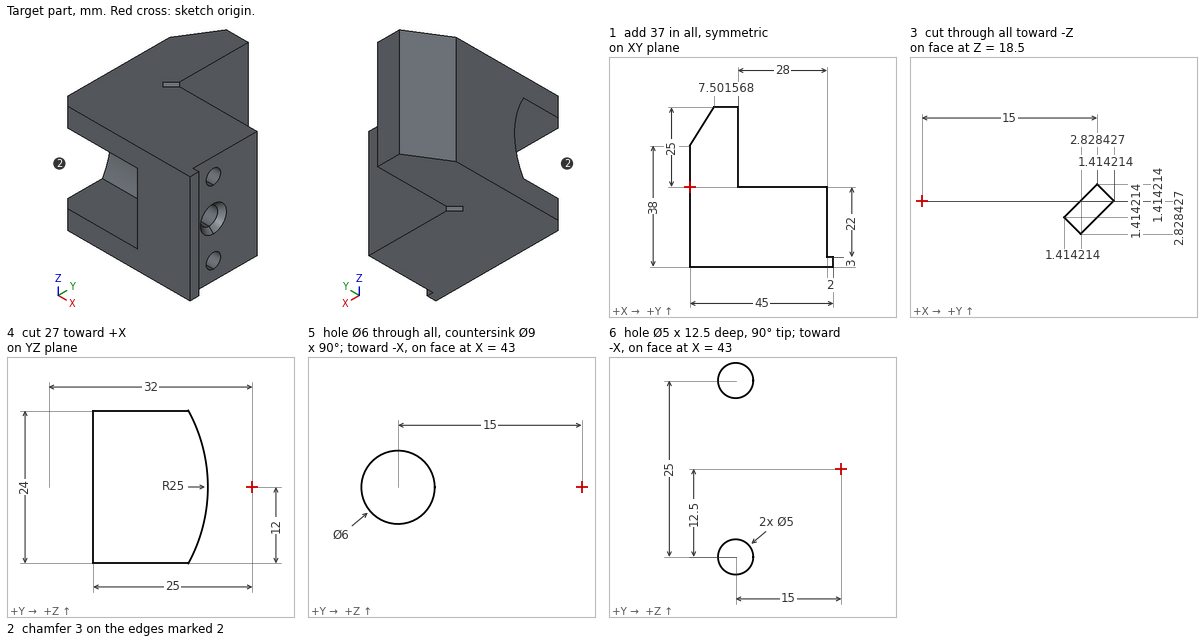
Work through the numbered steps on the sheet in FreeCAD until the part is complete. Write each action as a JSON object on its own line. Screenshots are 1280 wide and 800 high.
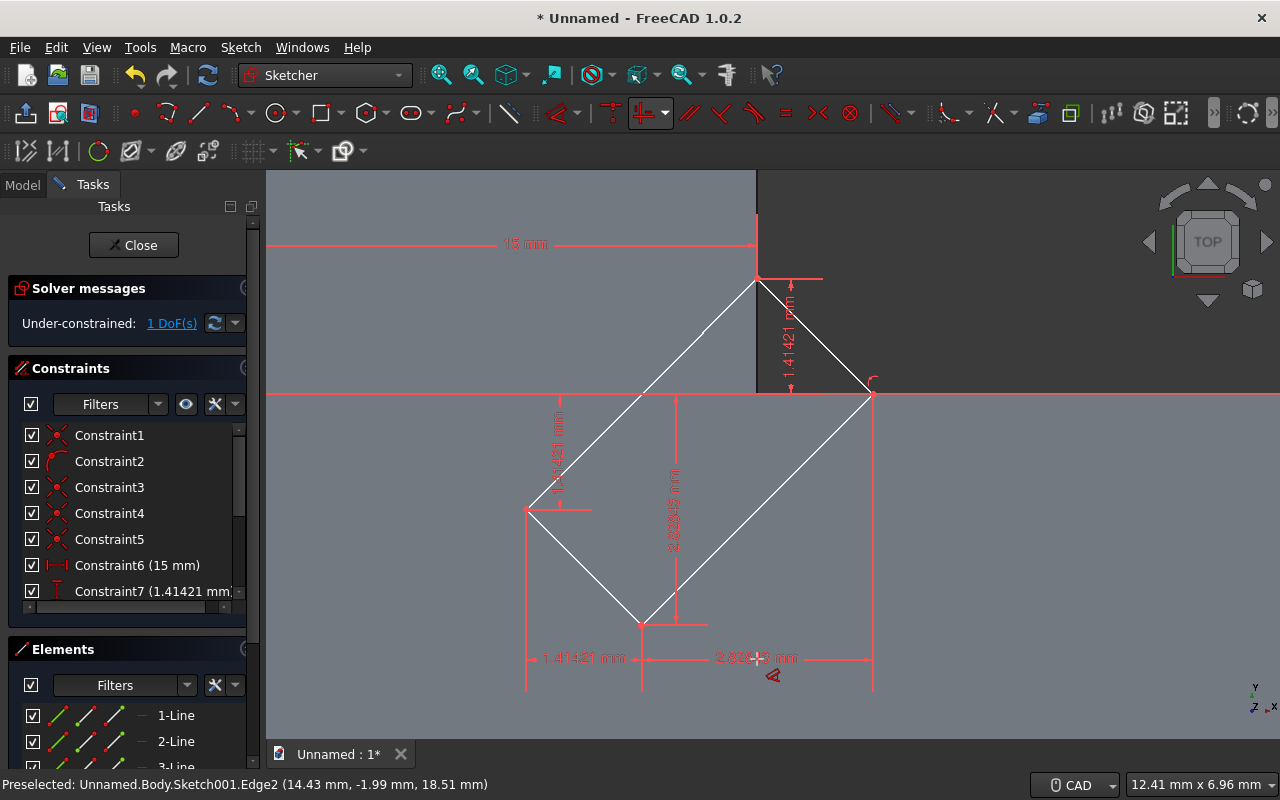
{"action": "left_click", "coordinate": [838, 360]}
{"action": "left_click", "coordinate": [815, 245]}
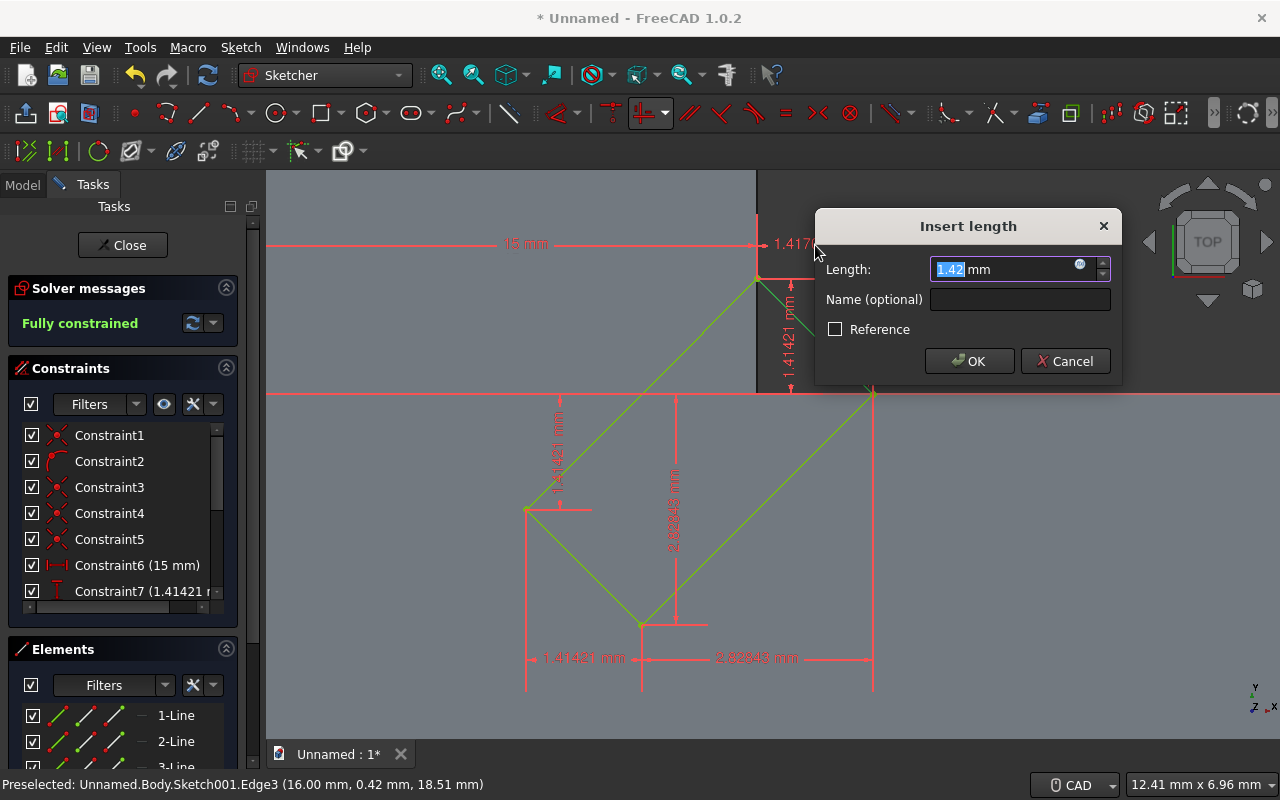
{"action": "type", "text": "1.414214"}
{"action": "key", "text": "Return"}
{"action": "key", "text": "Escape"}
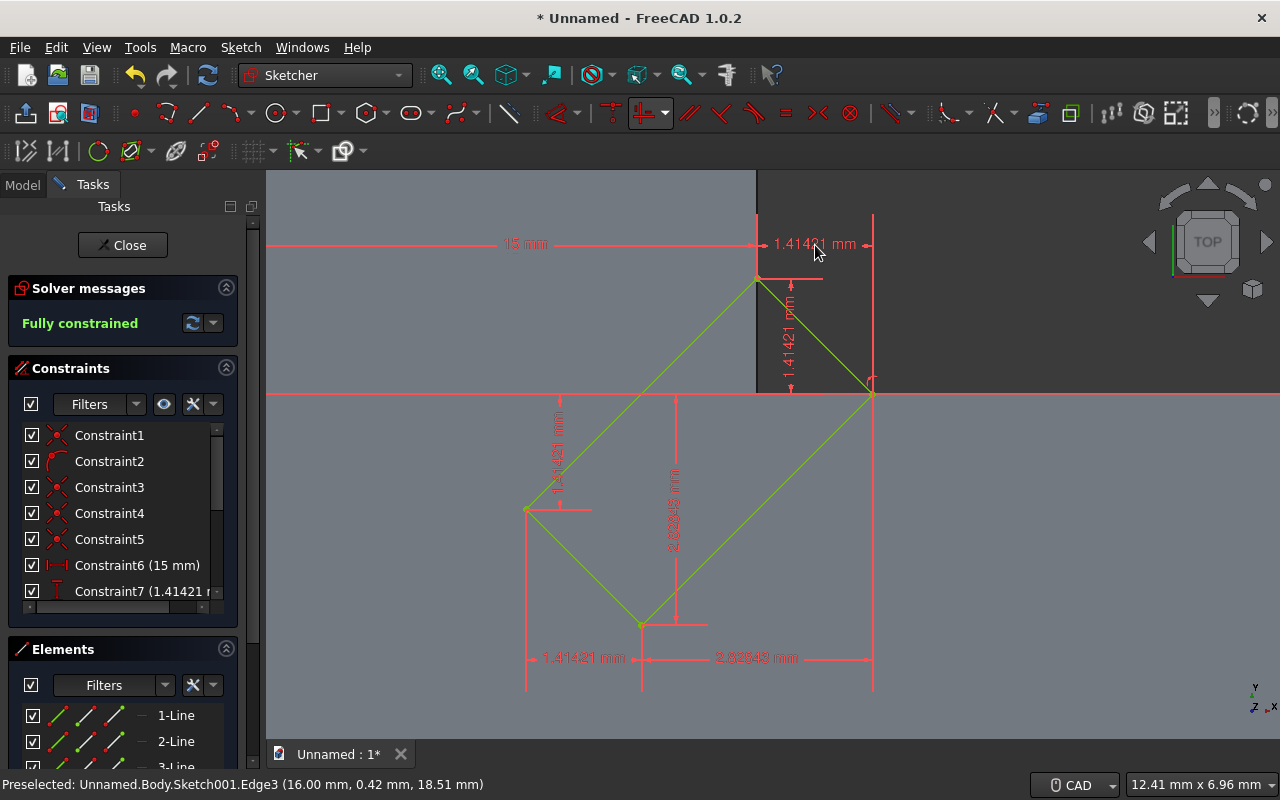
{"action": "left_click", "coordinate": [123, 245]}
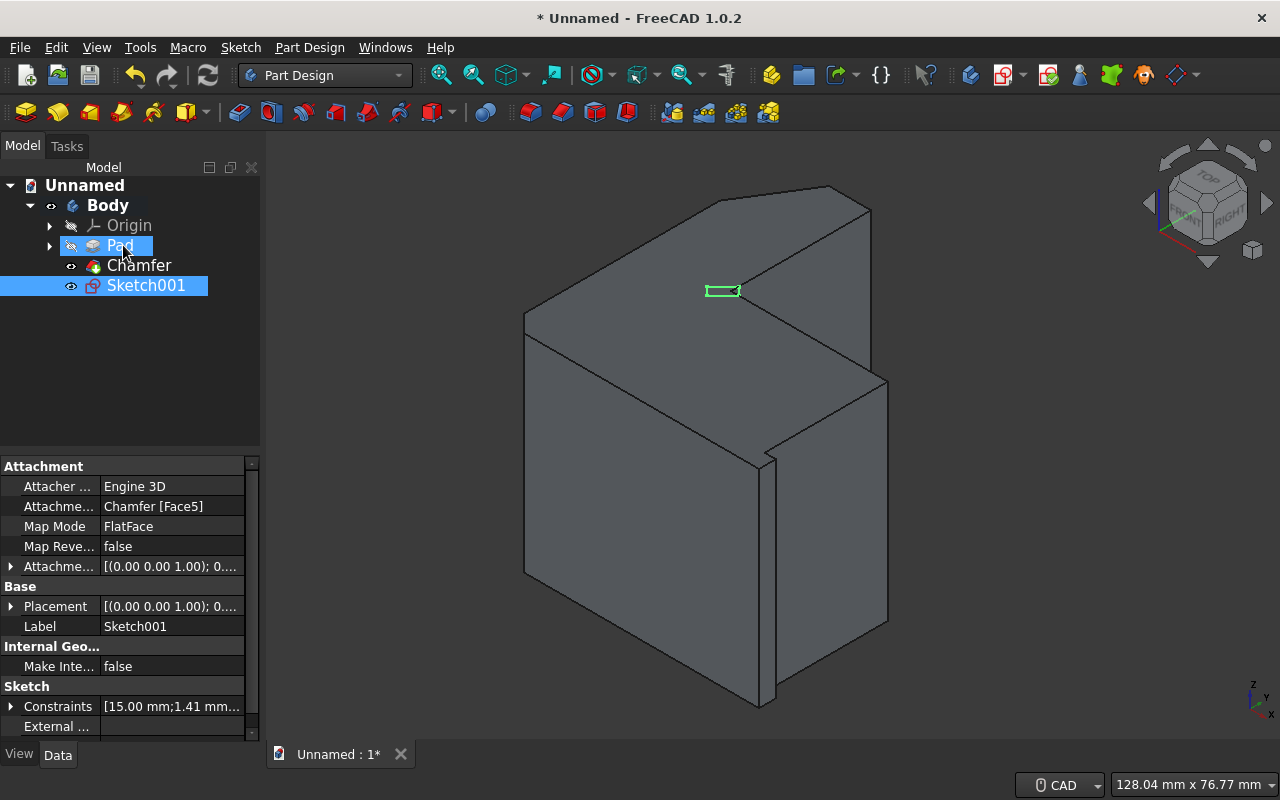
{"action": "left_click", "coordinate": [240, 112]}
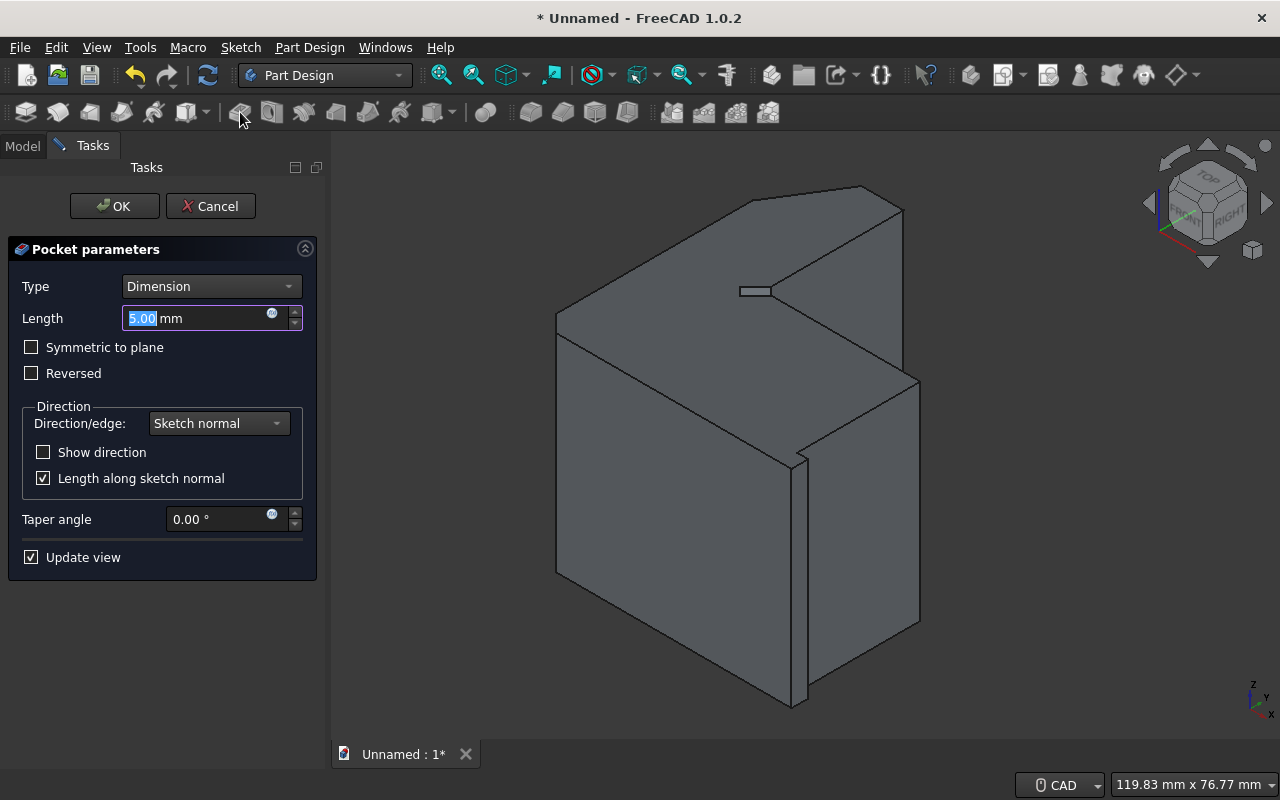
{"action": "left_click", "coordinate": [212, 286]}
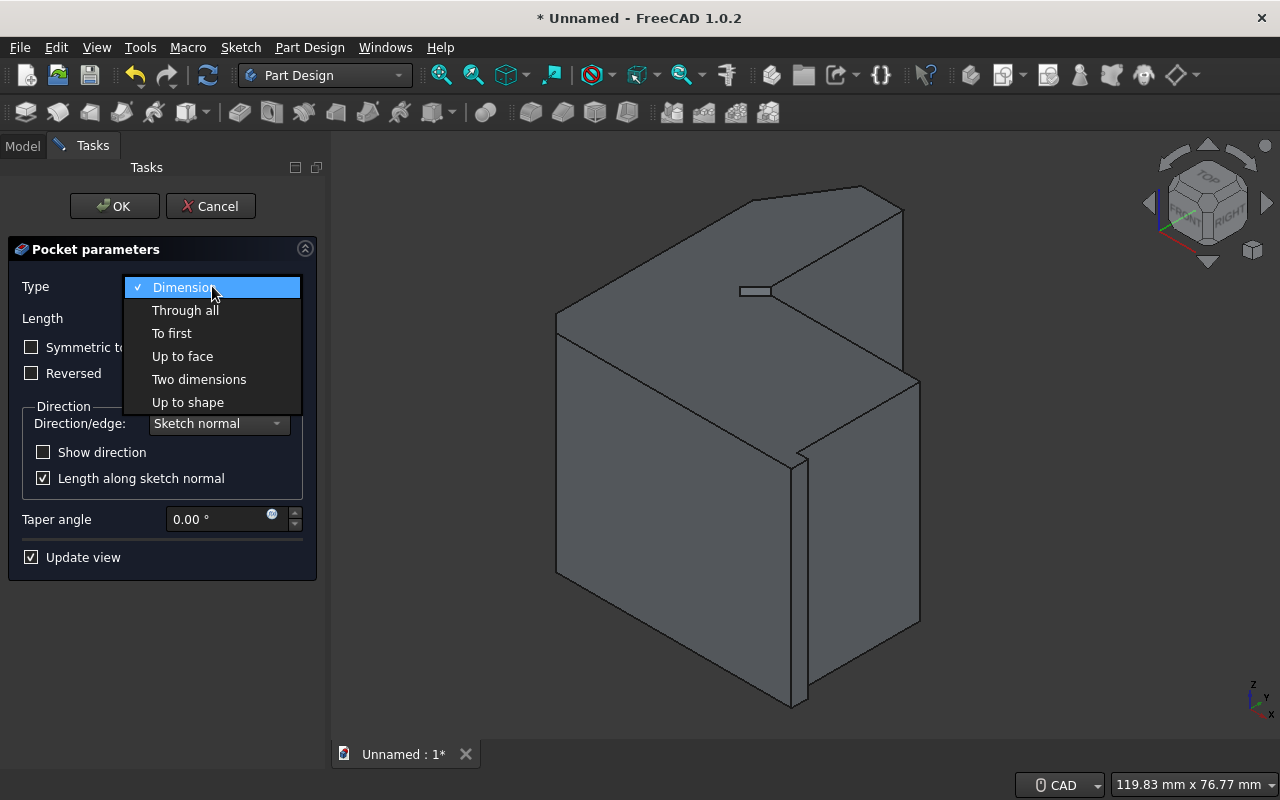
{"action": "left_click", "coordinate": [212, 310]}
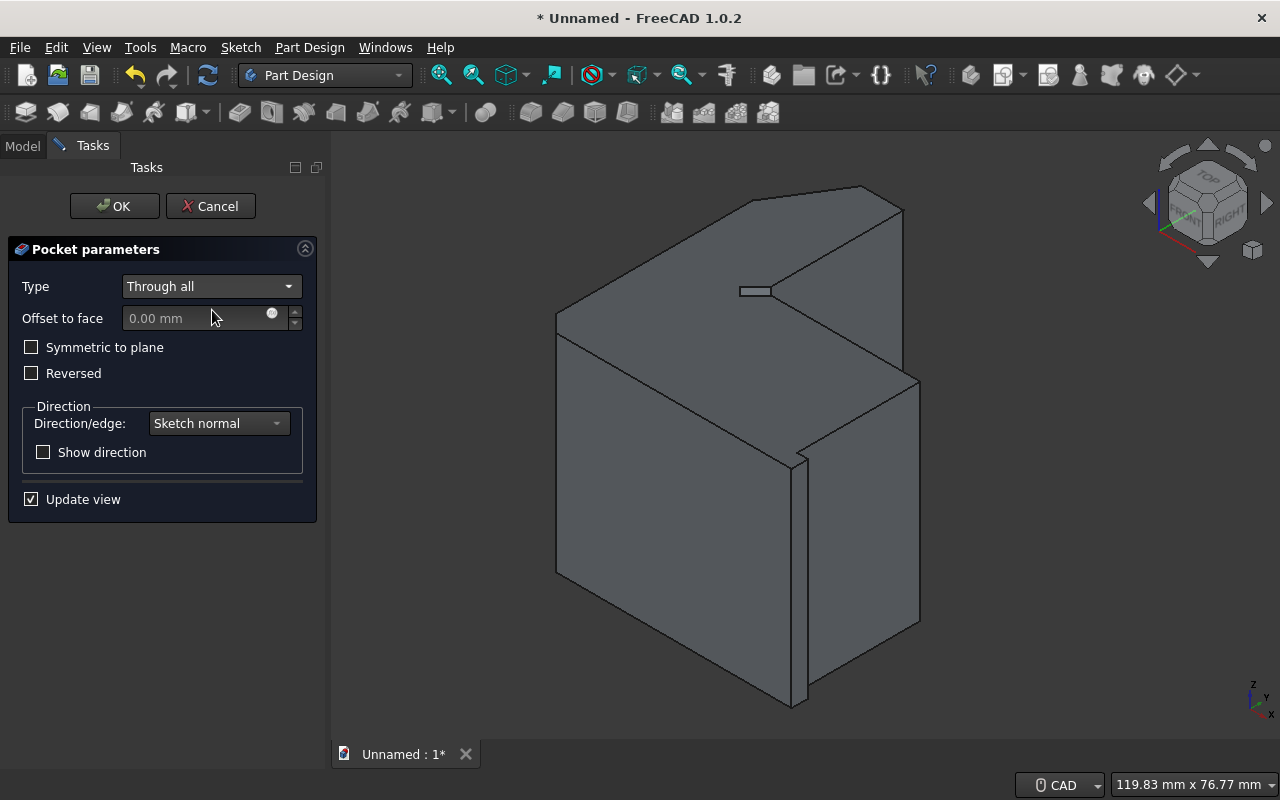
{"action": "left_click", "coordinate": [115, 206]}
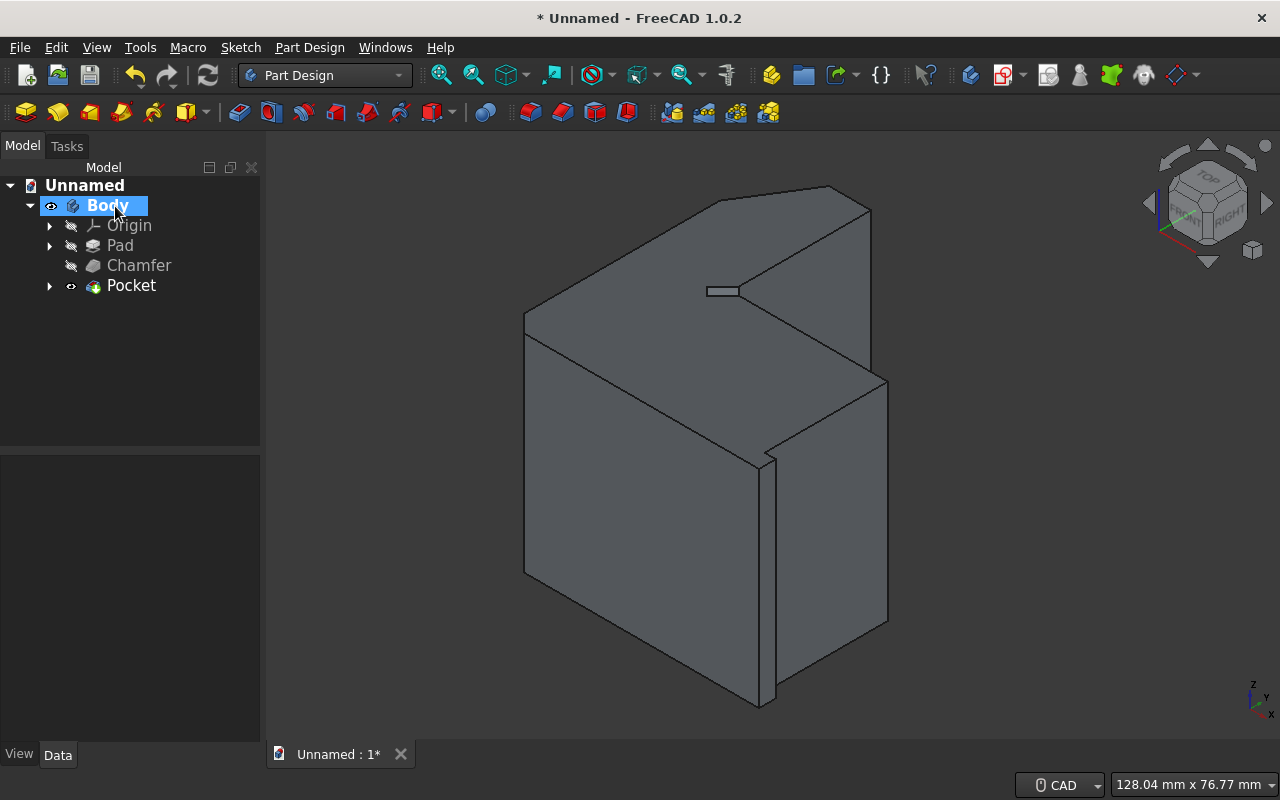
{"action": "left_click", "coordinate": [1004, 76]}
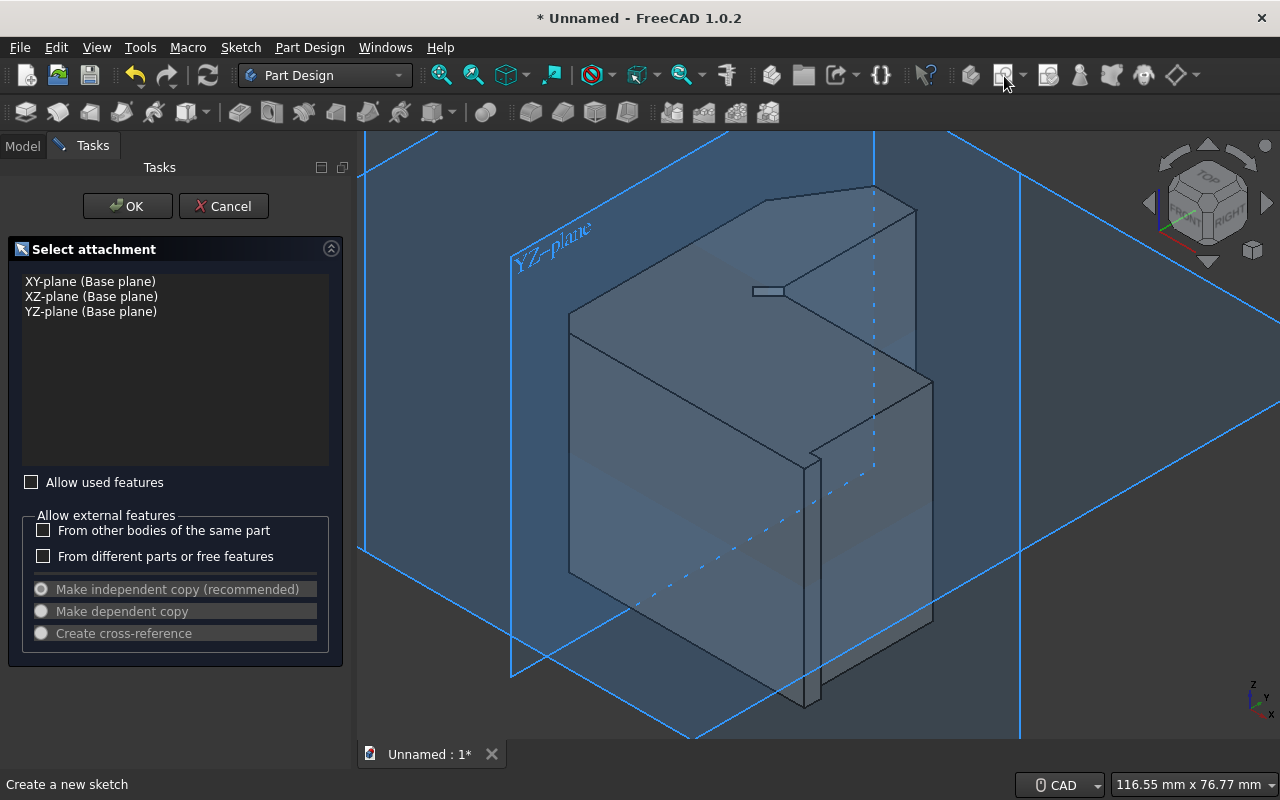
{"action": "left_click", "coordinate": [82, 312]}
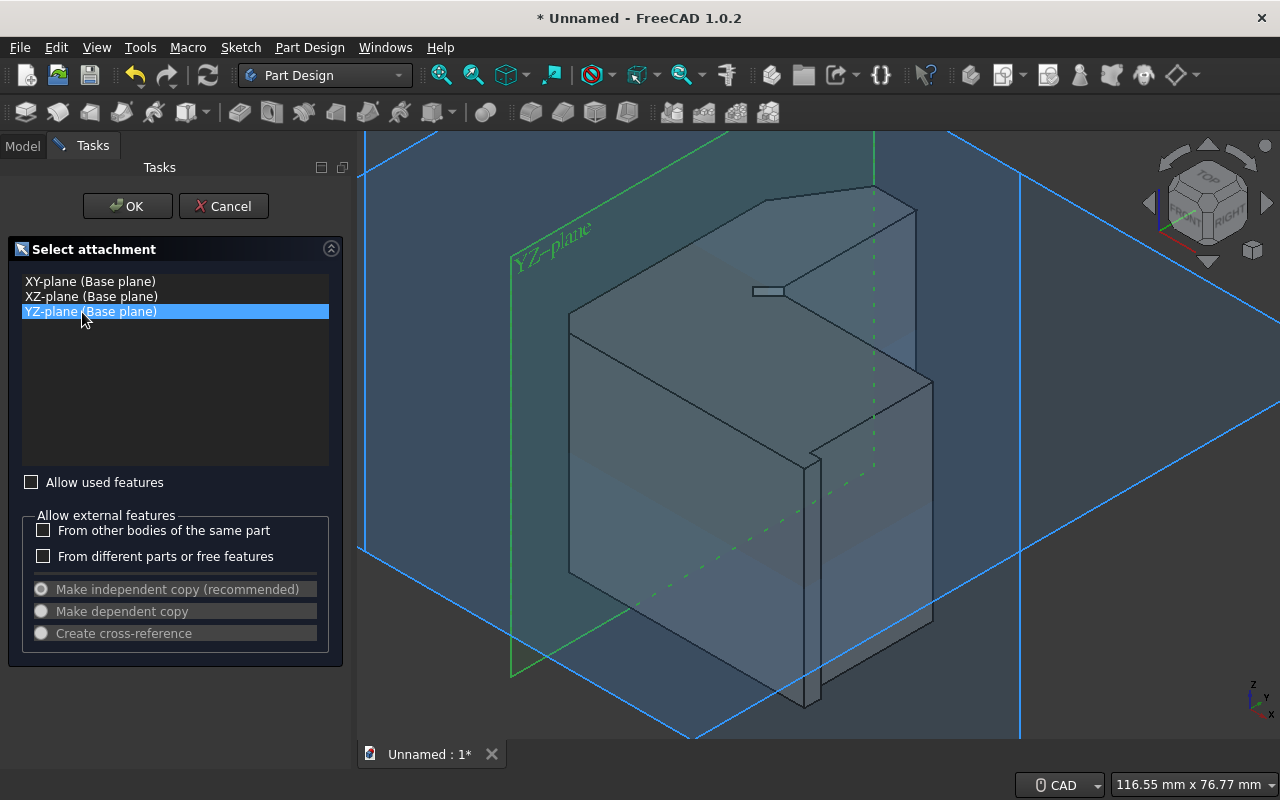
{"action": "left_click", "coordinate": [128, 206]}